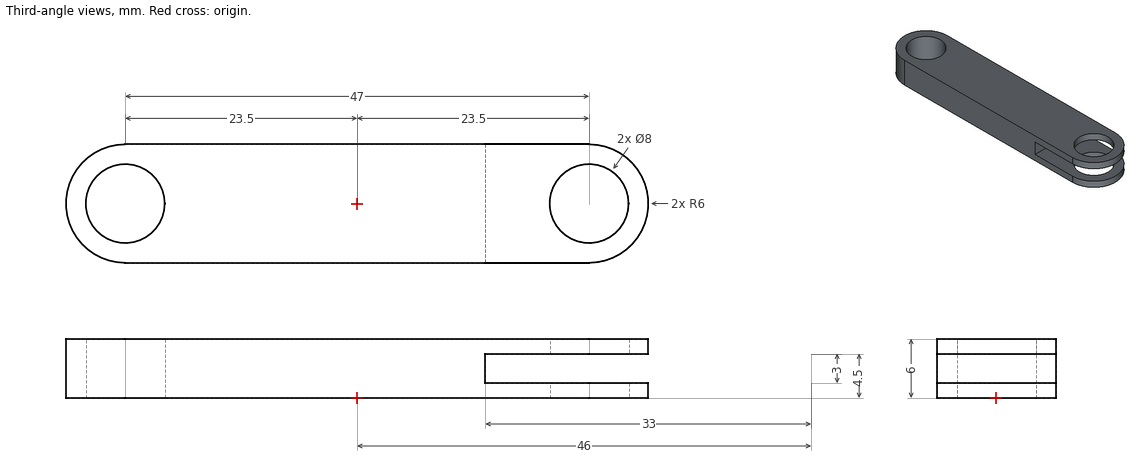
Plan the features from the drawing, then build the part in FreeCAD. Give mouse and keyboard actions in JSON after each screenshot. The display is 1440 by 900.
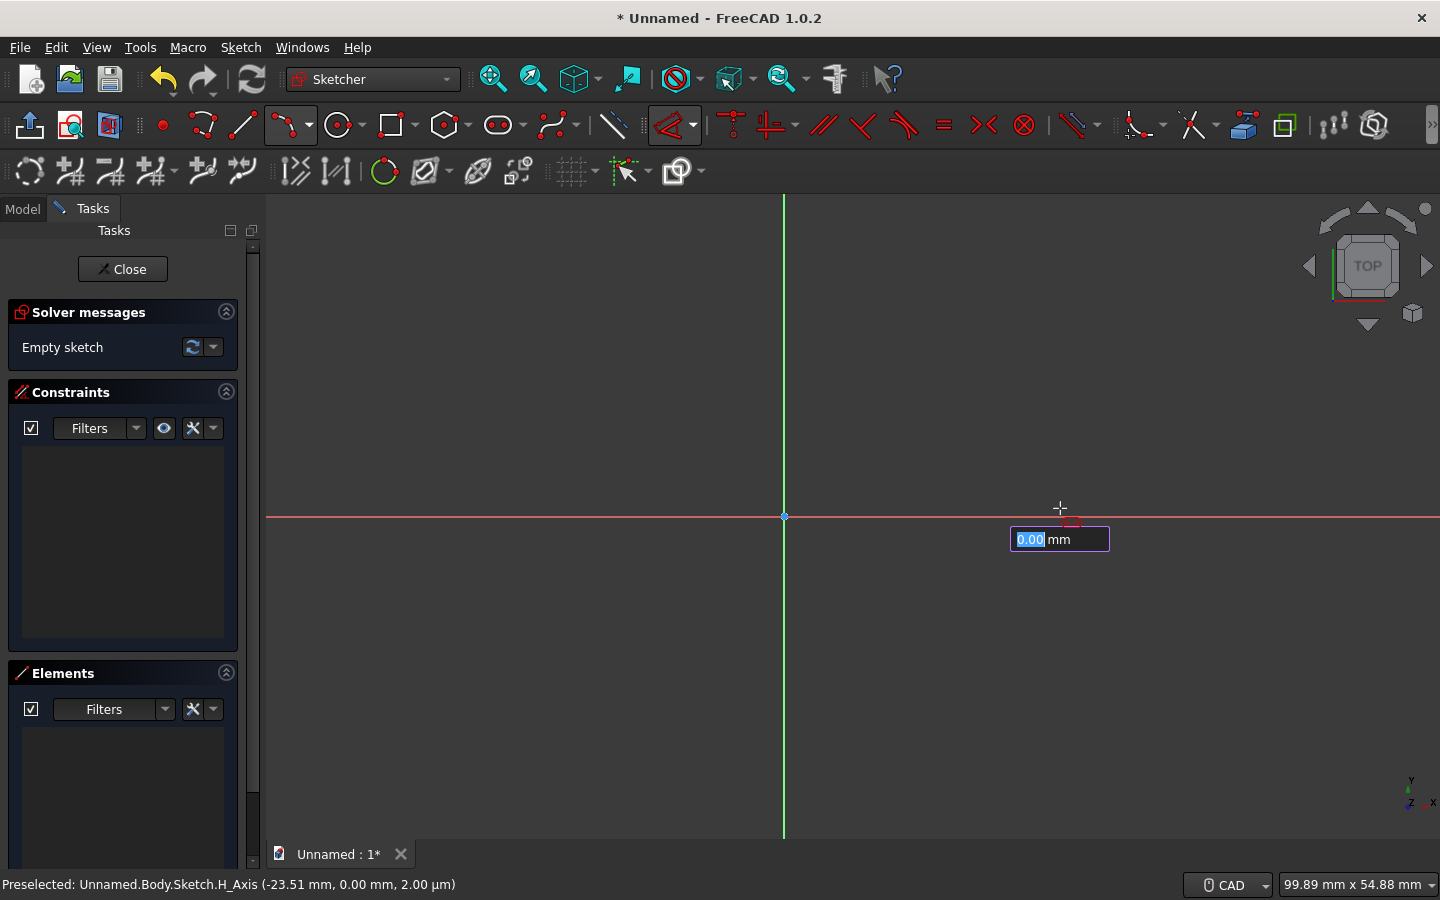
{"action": "left_click", "coordinate": [701, 587]}
{"action": "key", "text": "Escape"}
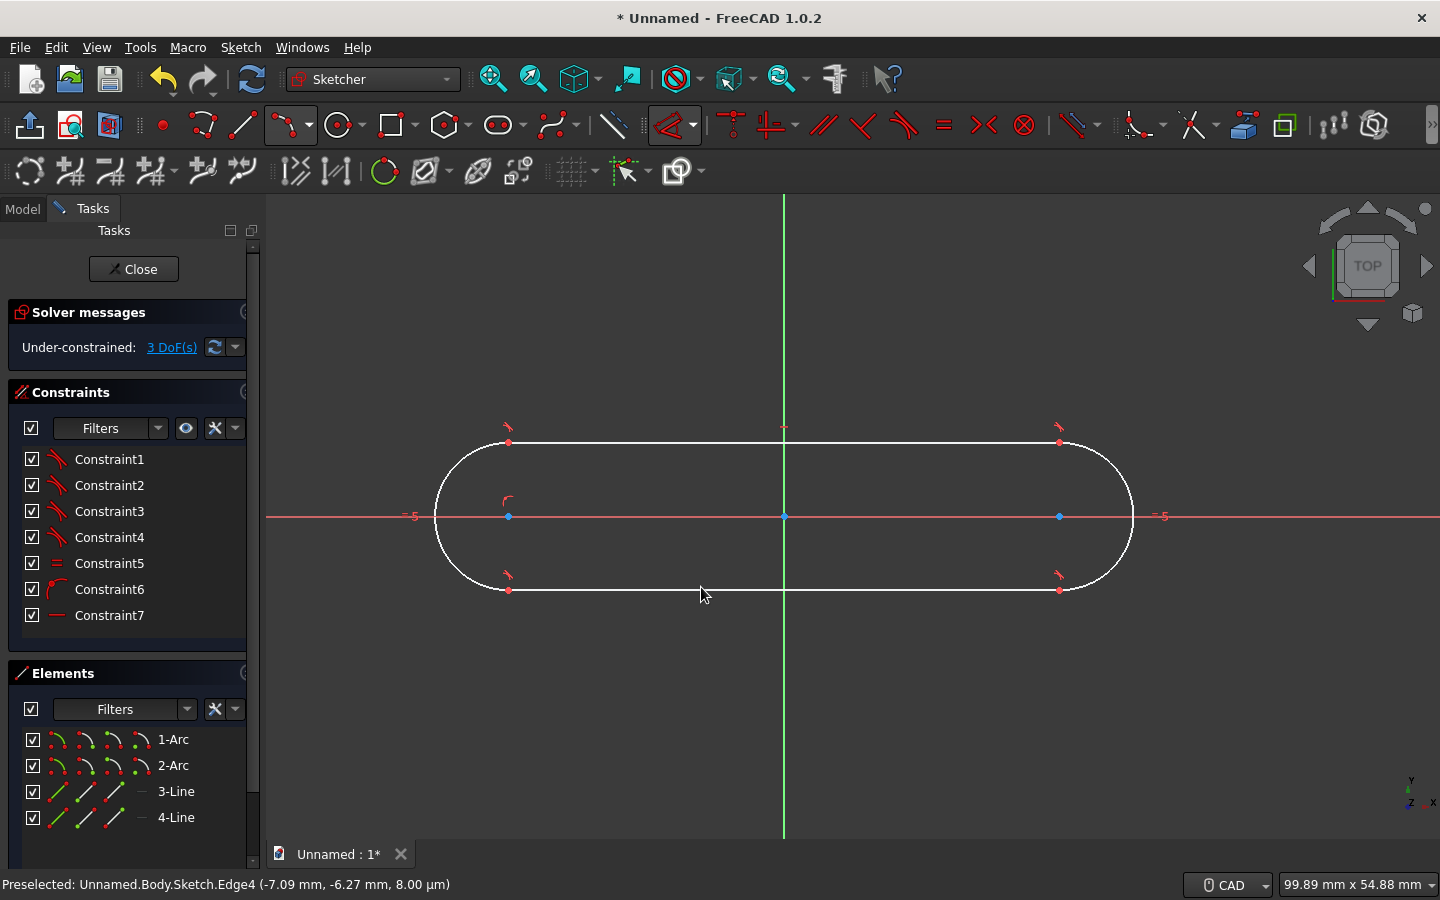
{"action": "left_click", "coordinate": [449, 473]}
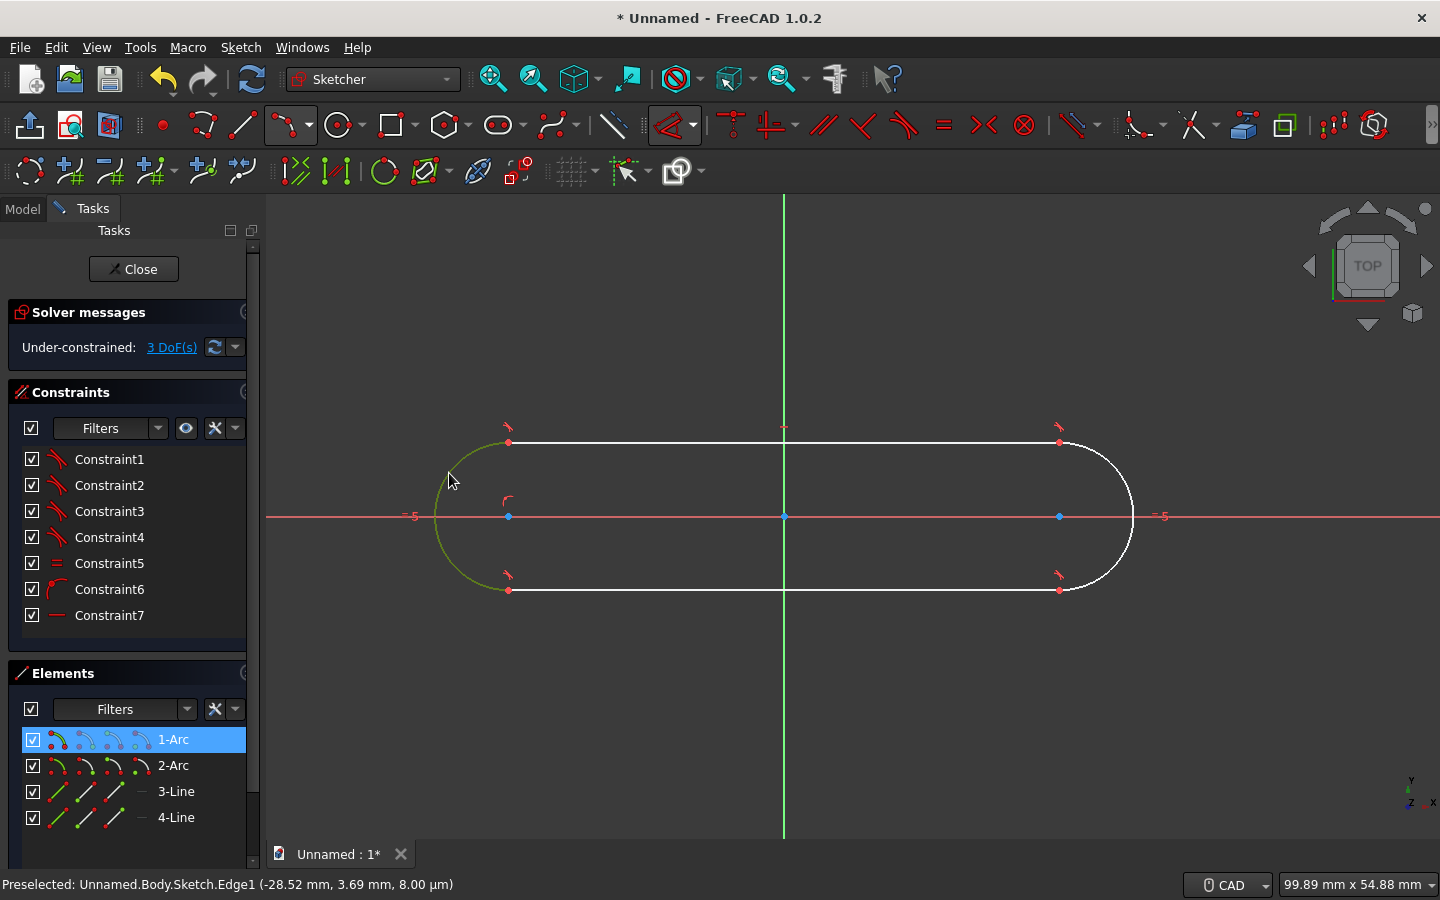
{"action": "key", "text": "k r"}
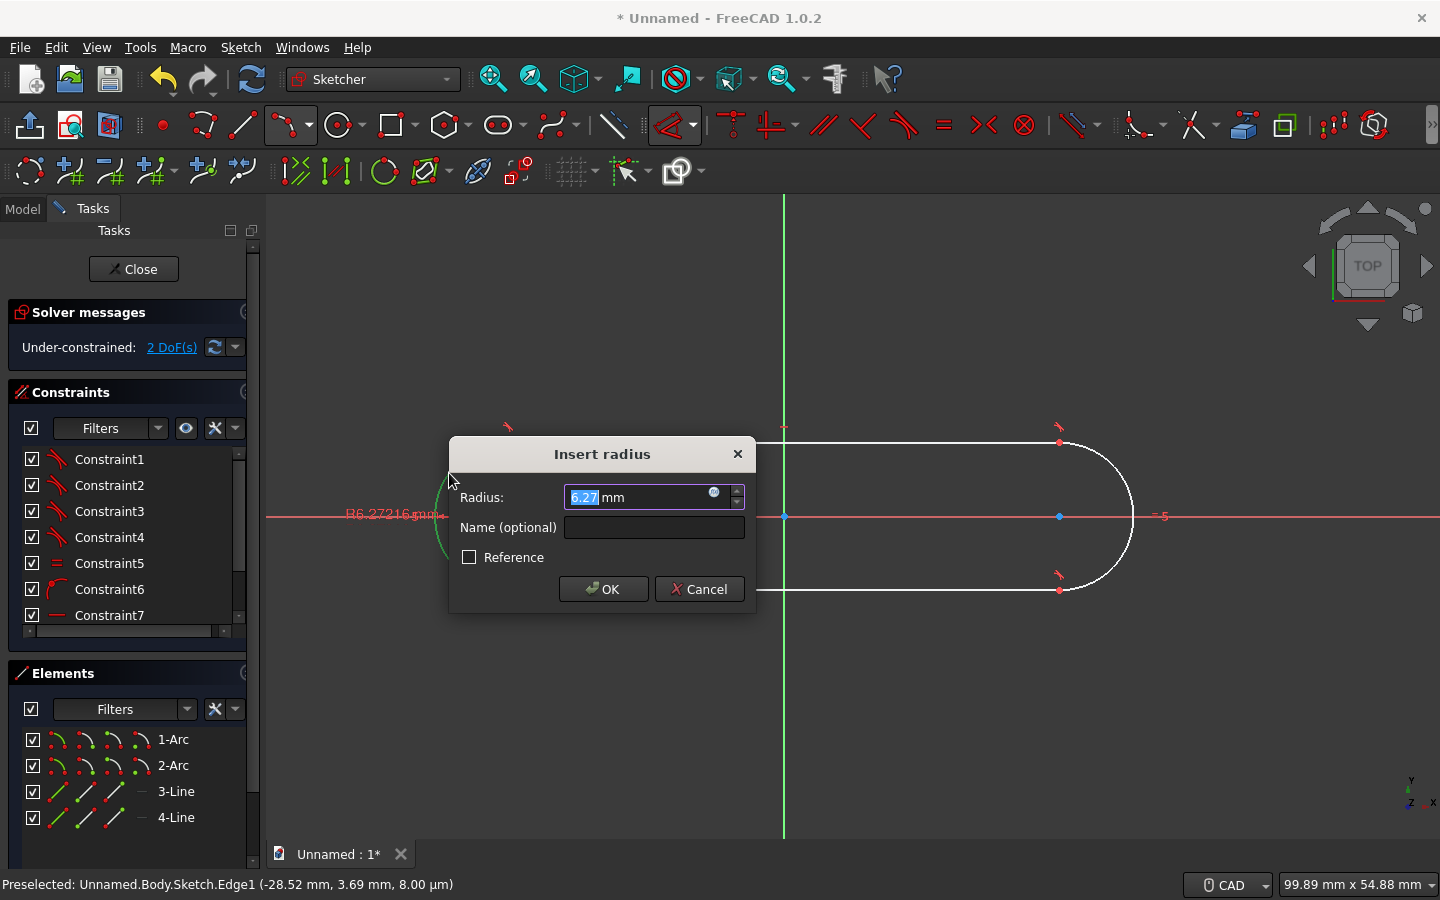
{"action": "type", "text": "6"}
{"action": "key", "text": "Return"}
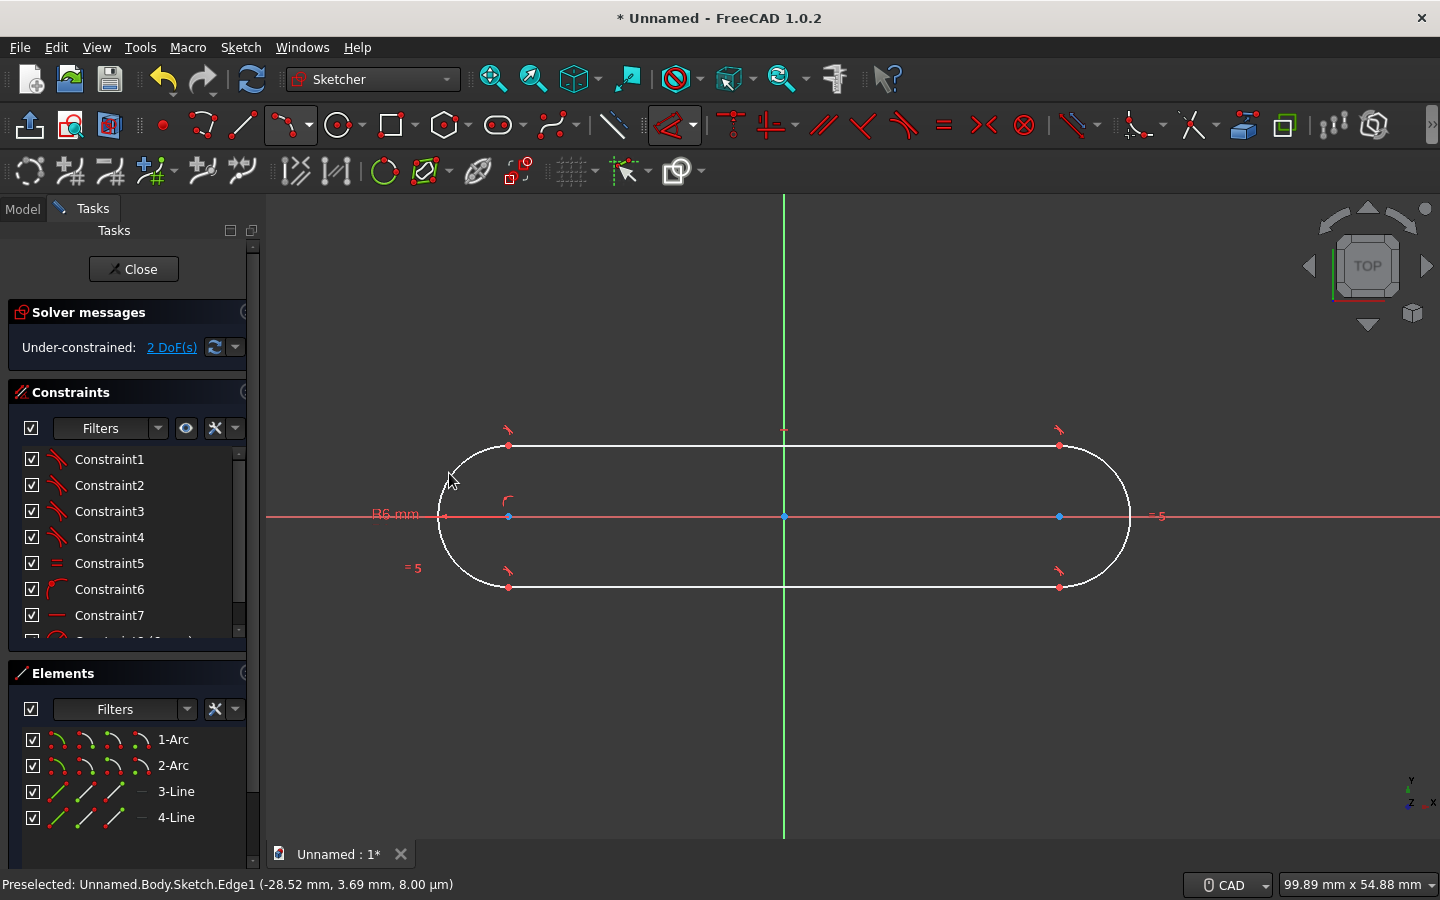
{"action": "left_click", "coordinate": [674, 446]}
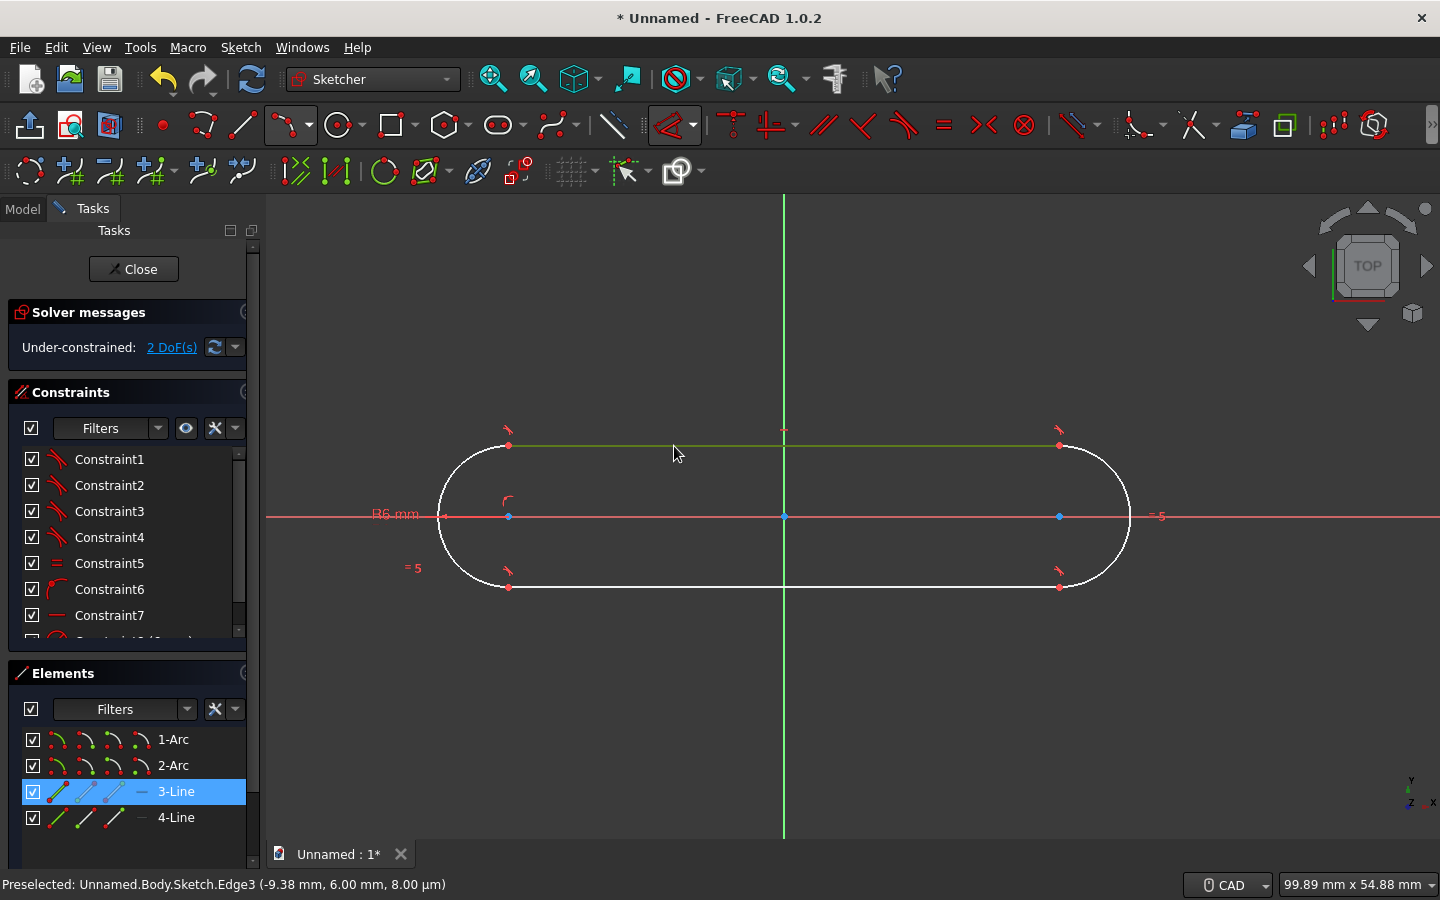
{"action": "key", "text": "l"}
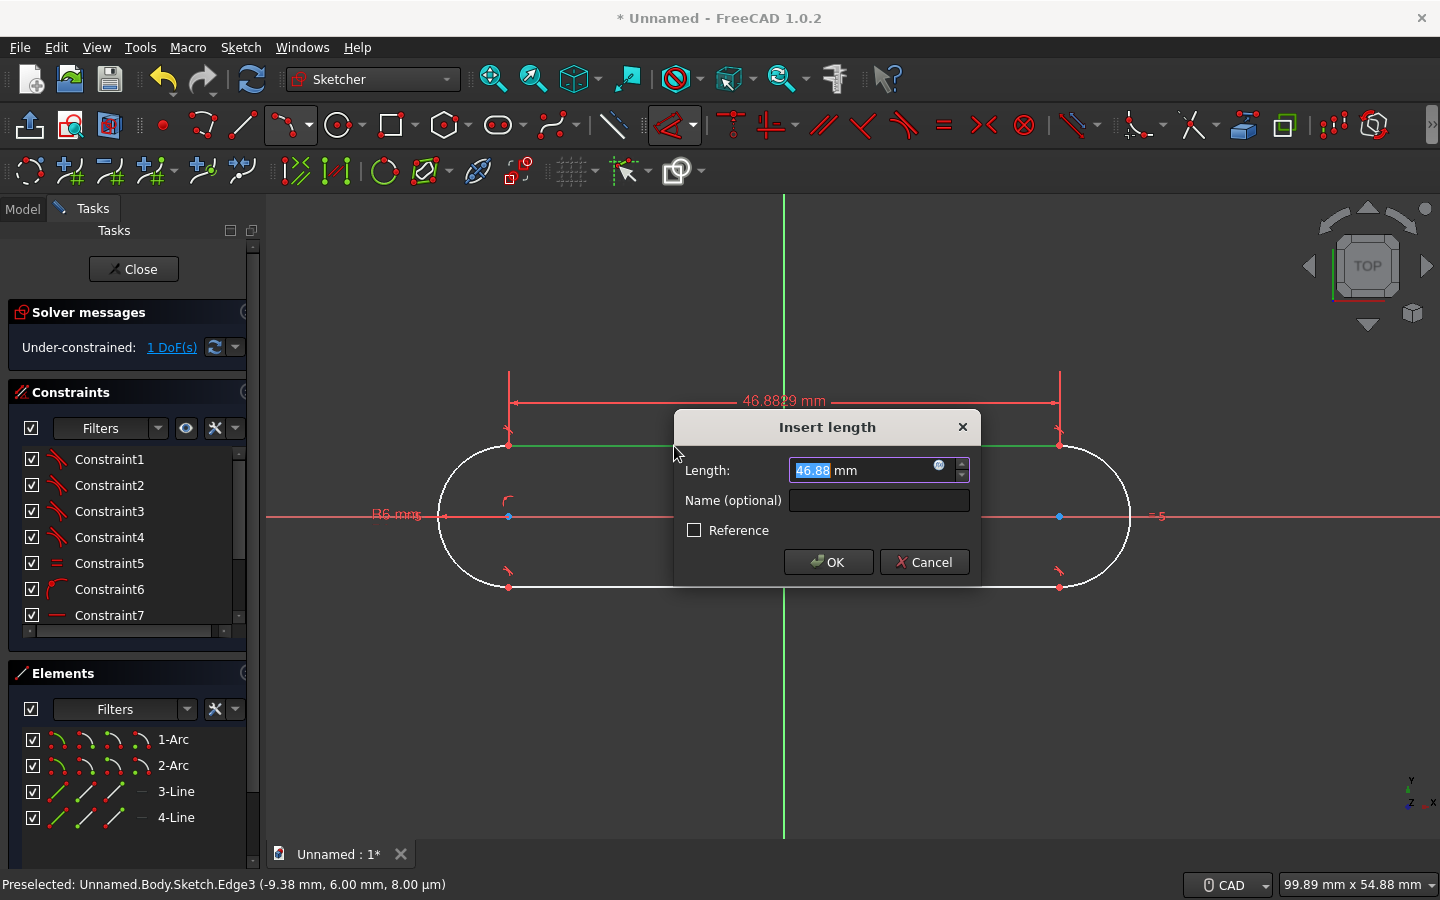
{"action": "type", "text": "47"}
{"action": "key", "text": "Return"}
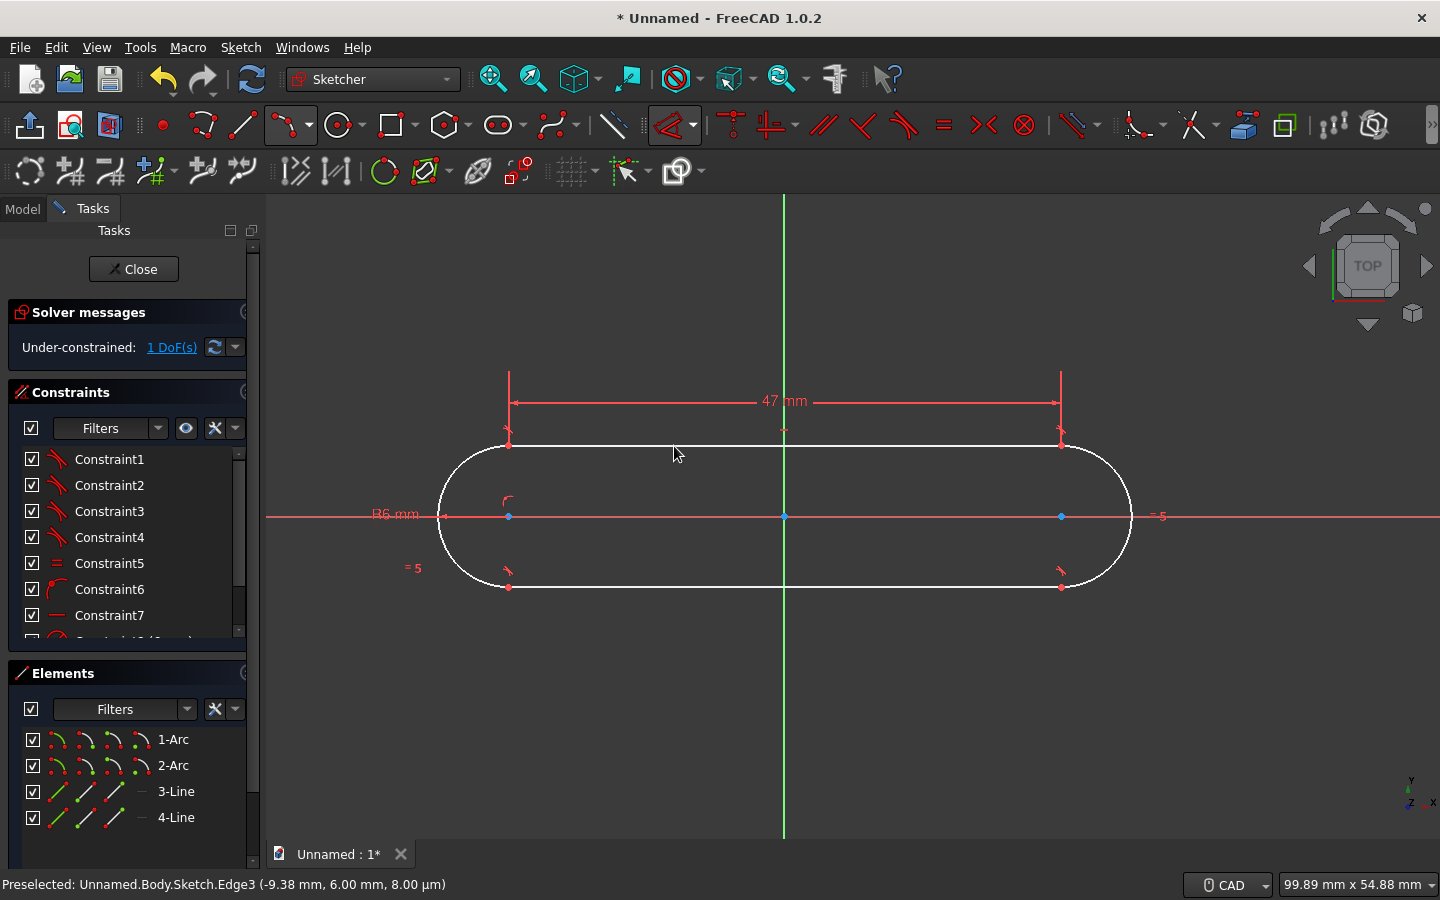
{"action": "left_click", "coordinate": [509, 446]}